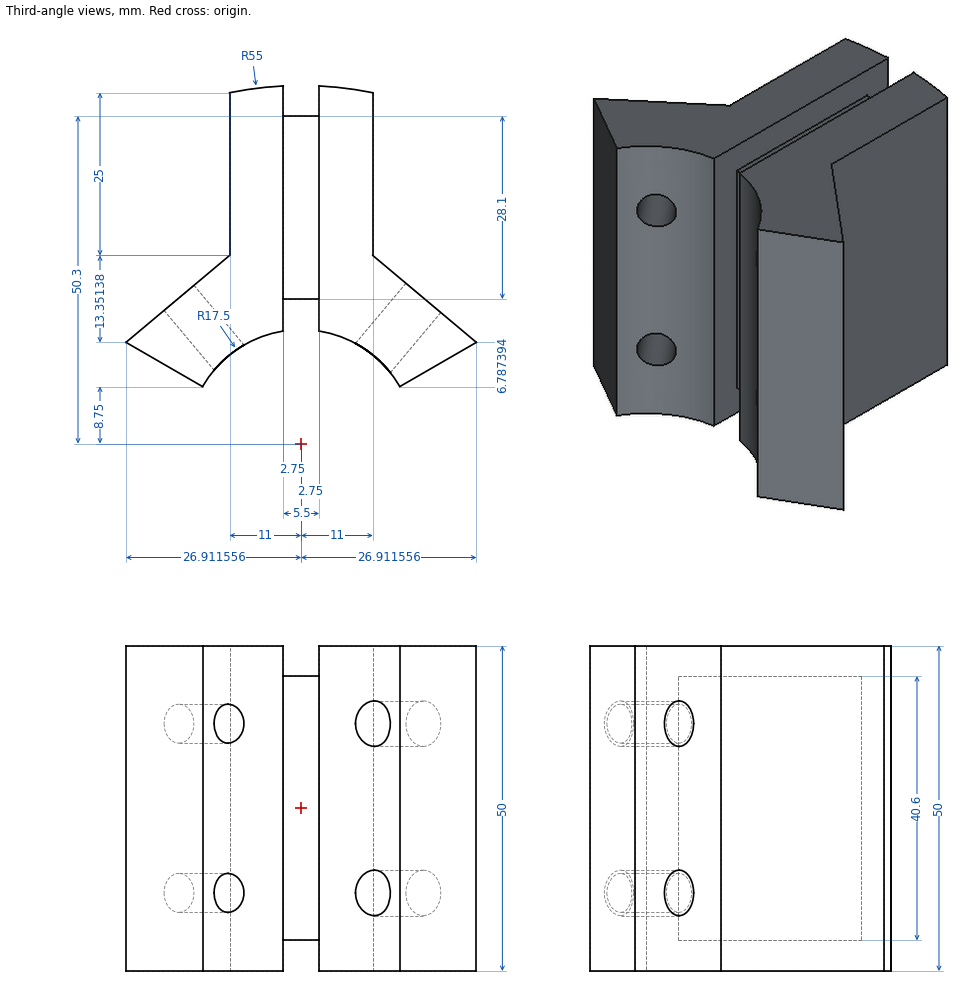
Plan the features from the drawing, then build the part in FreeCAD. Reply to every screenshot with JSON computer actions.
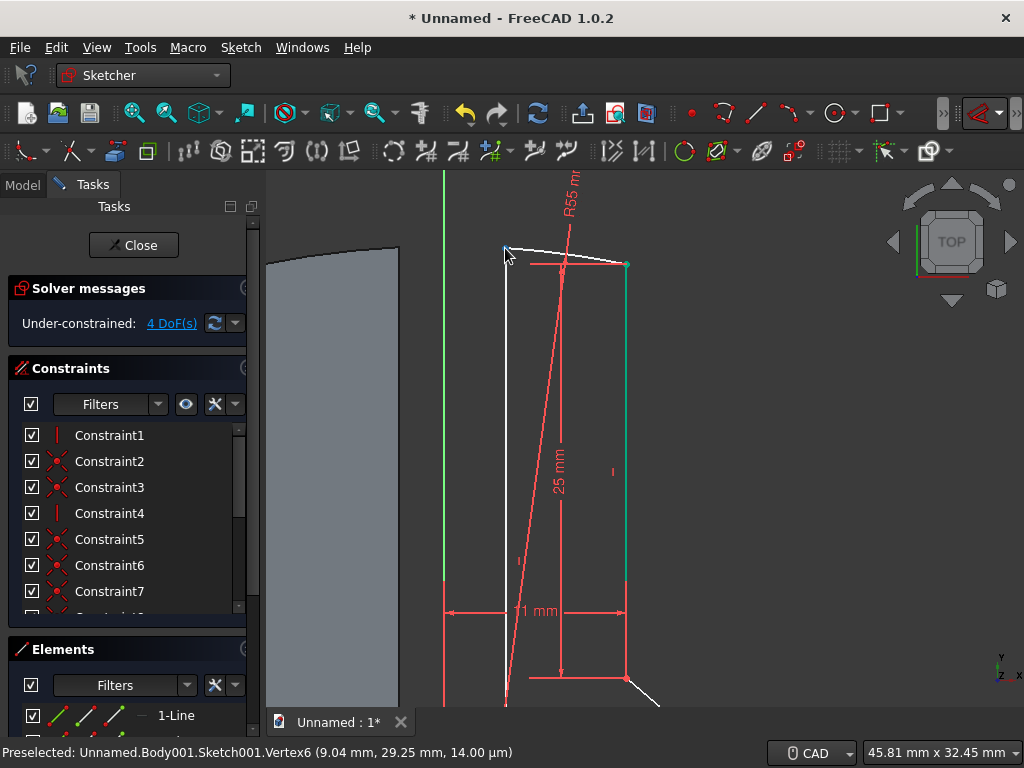
{"action": "left_click", "coordinate": [506, 248]}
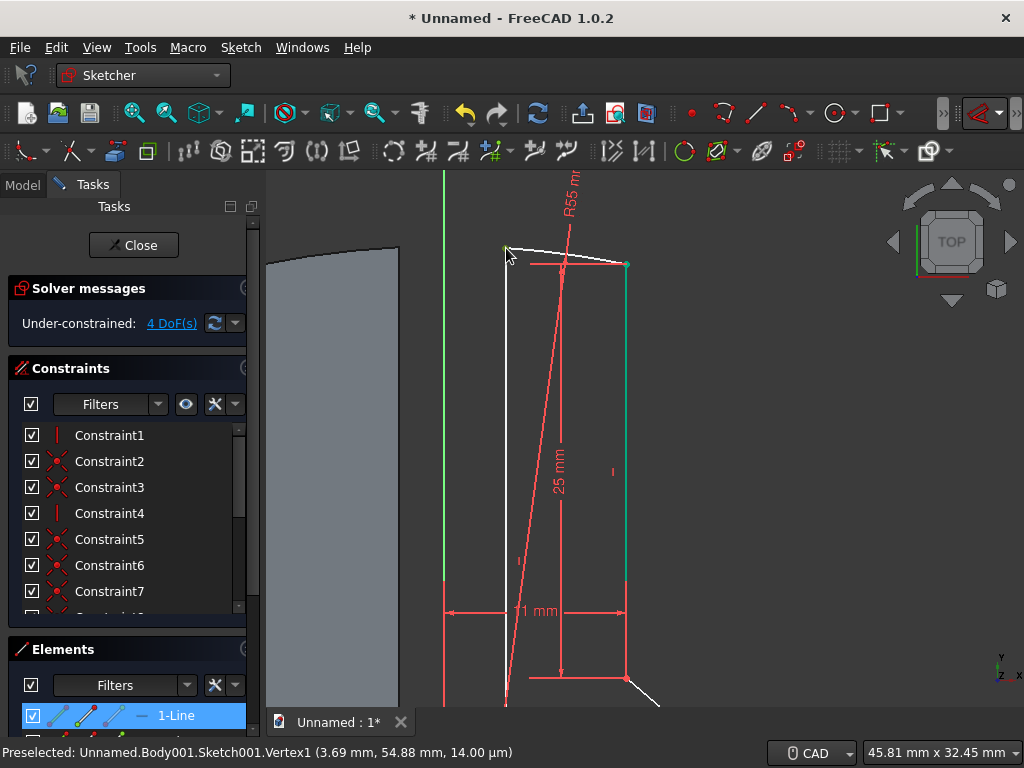
{"action": "key", "text": "l"}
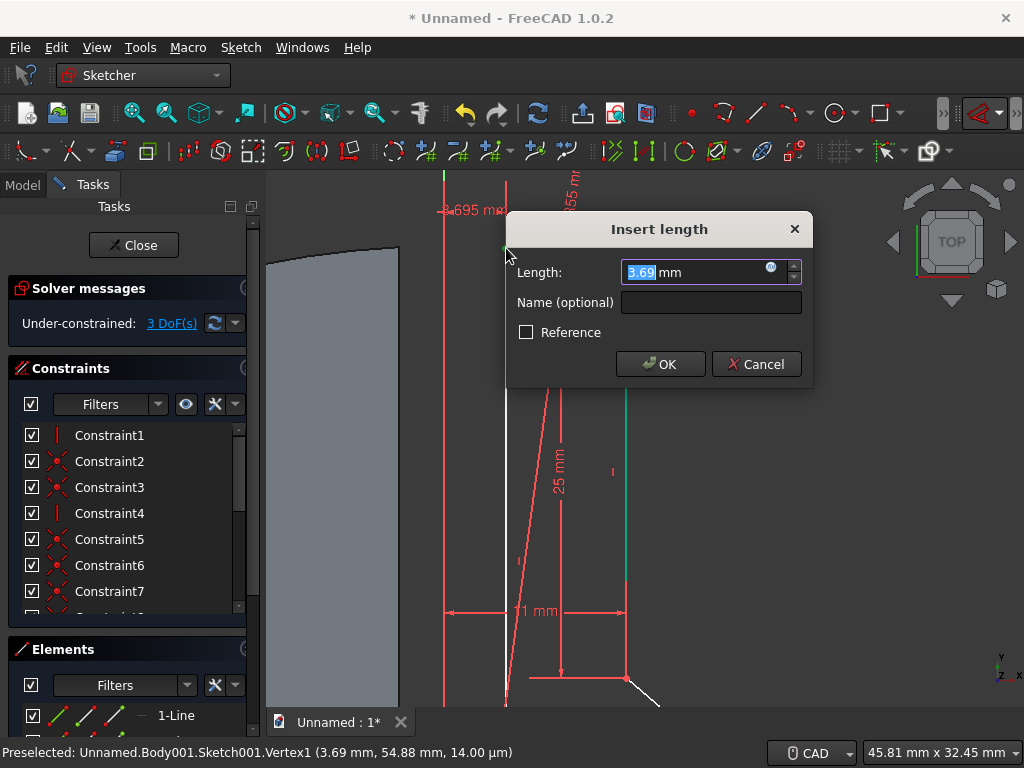
{"action": "type", "text": "2.75"}
{"action": "key", "text": "Return"}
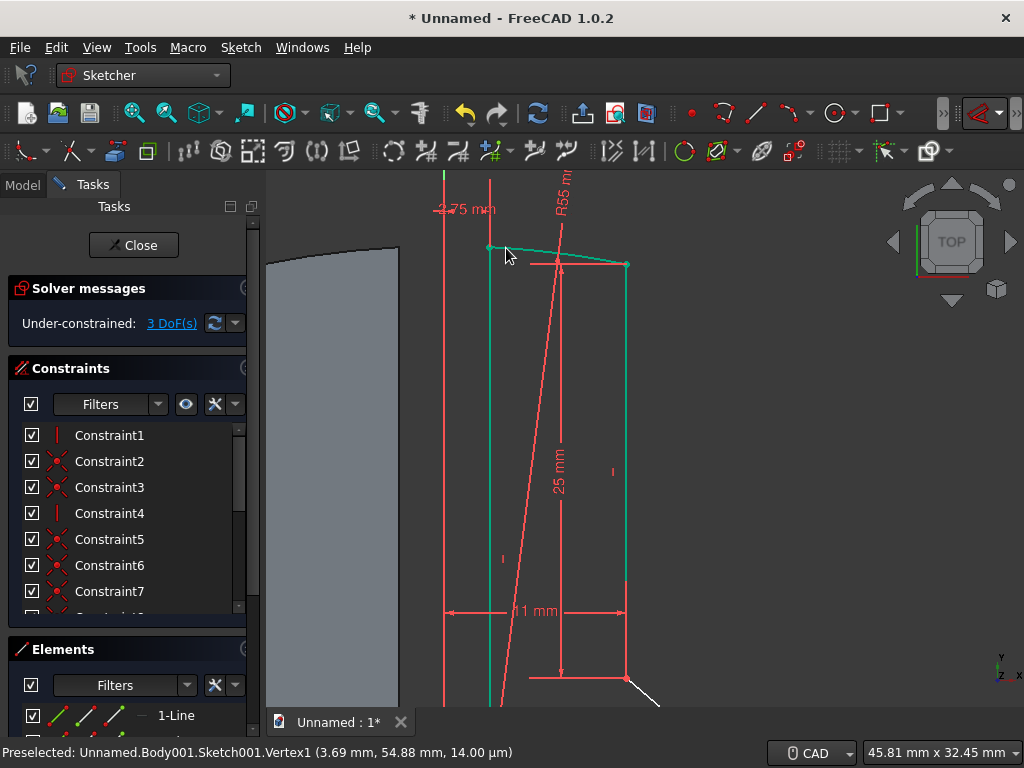
{"action": "scroll", "coordinate": [524, 285], "scroll_direction": "down", "scroll_amount": 5}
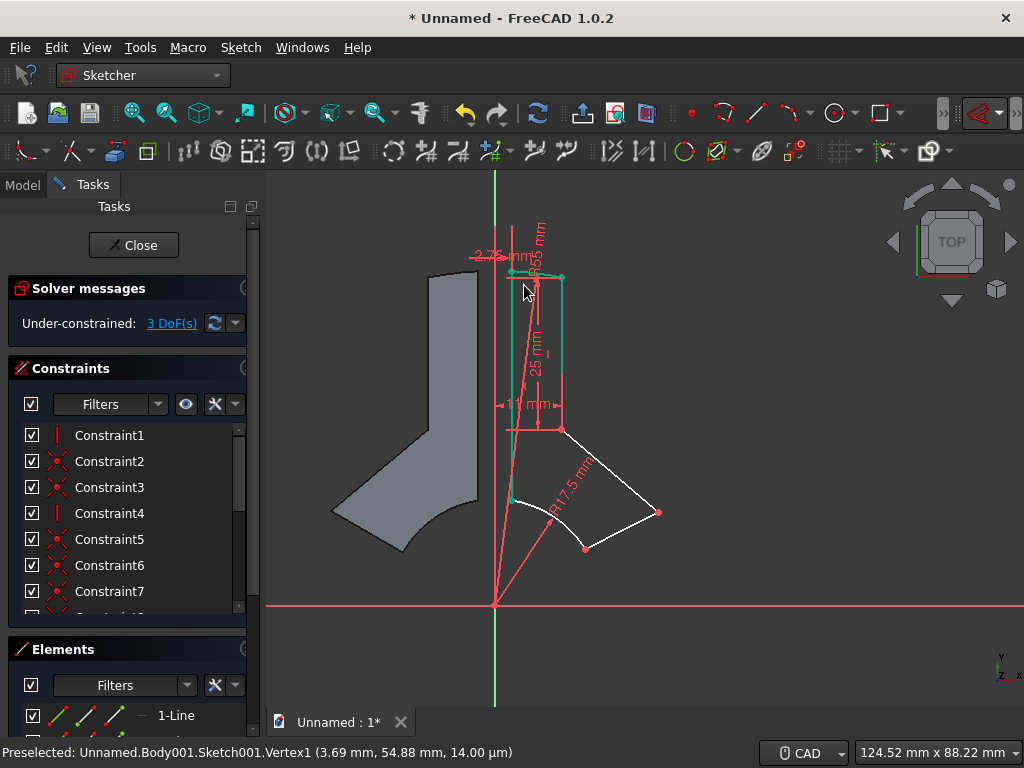
{"action": "left_click", "coordinate": [585, 549]}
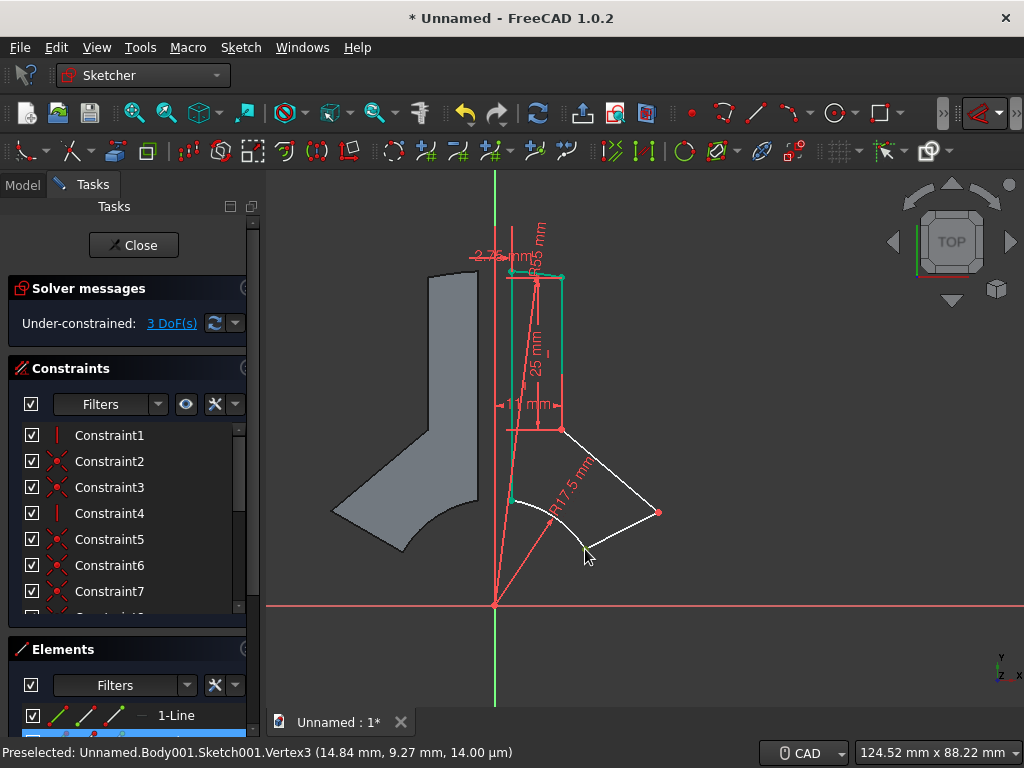
{"action": "left_click", "coordinate": [1002, 114]}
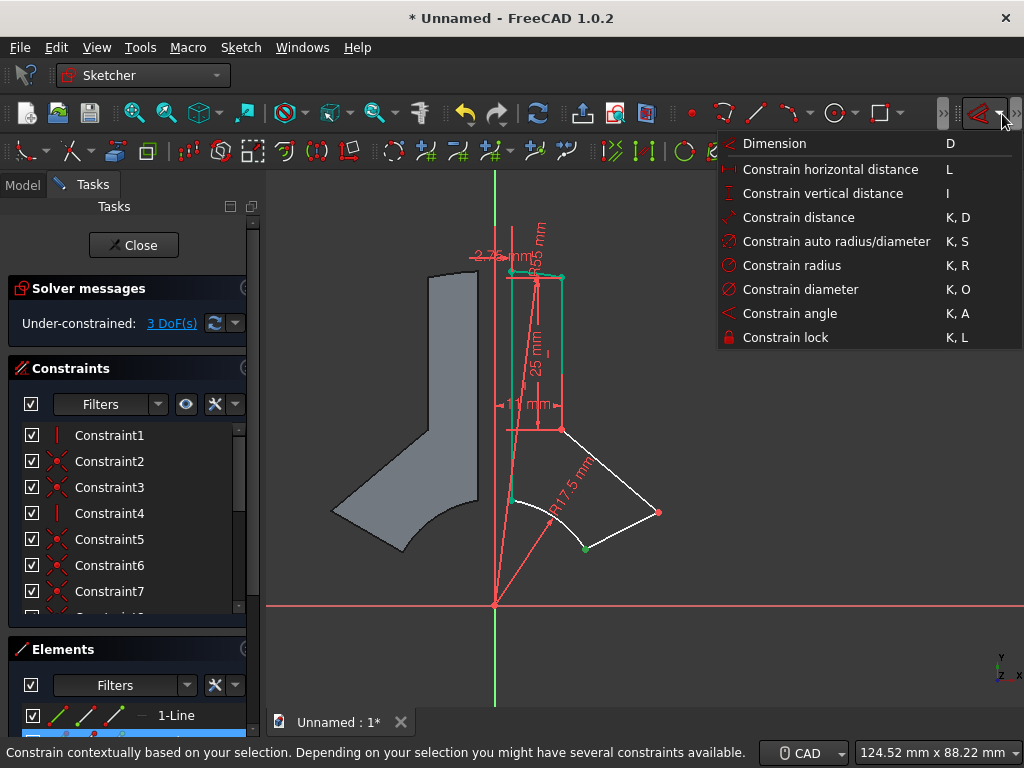
{"action": "left_click", "coordinate": [870, 193]}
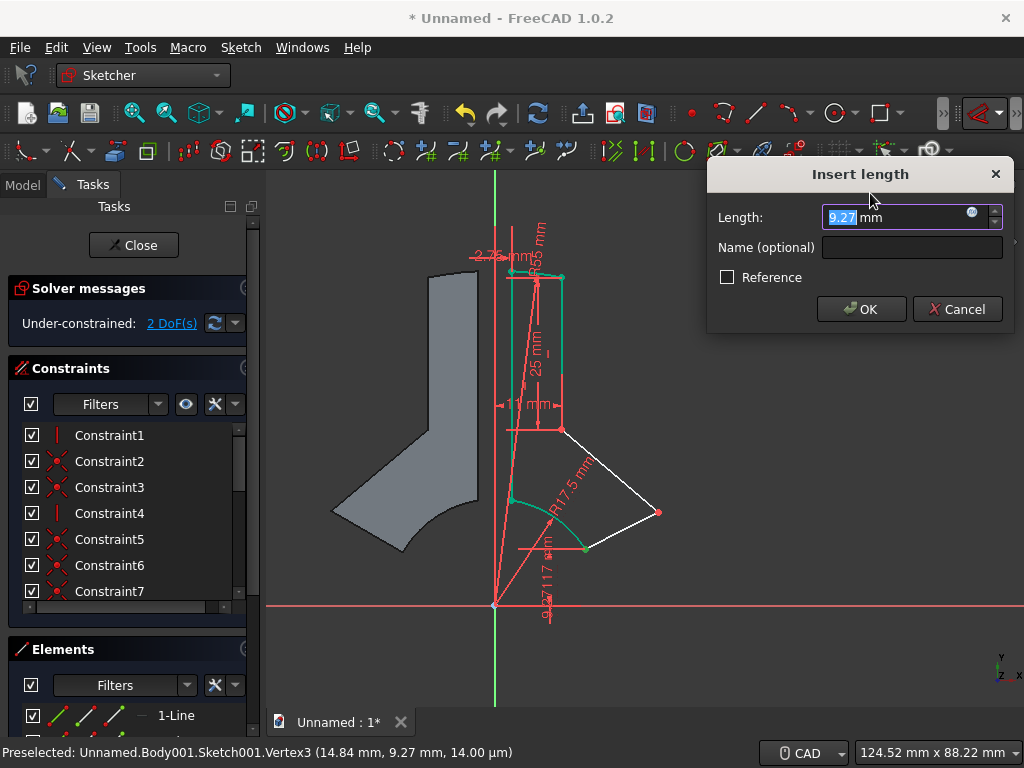
{"action": "type", "text": "8.75"}
{"action": "key", "text": "Return"}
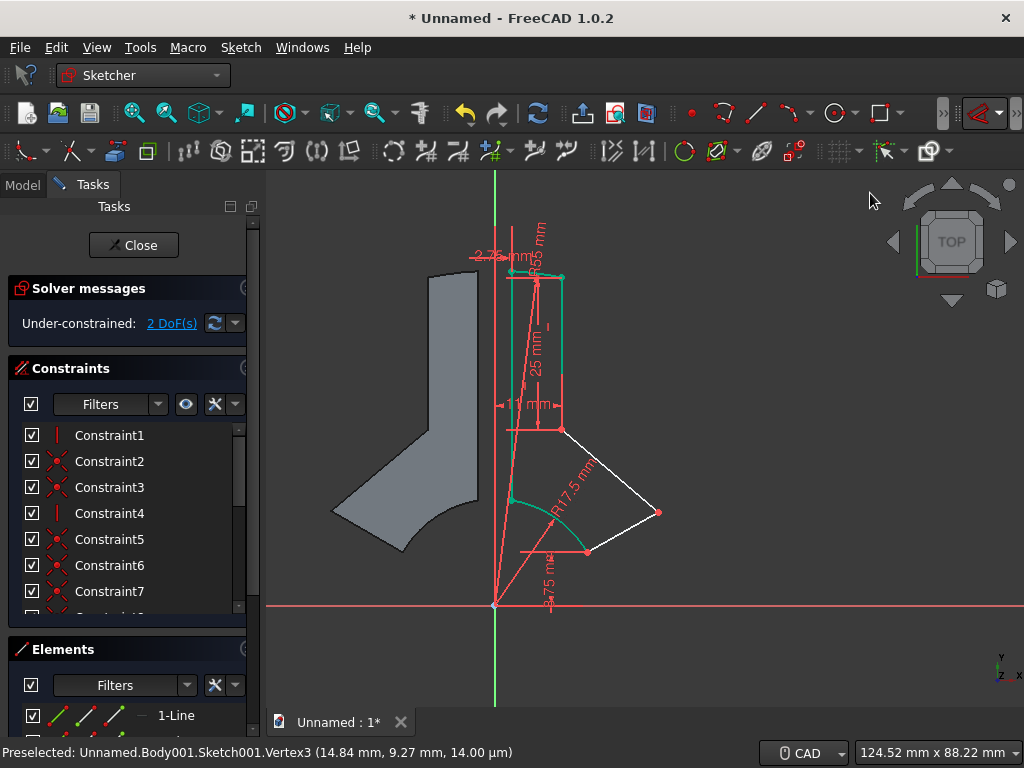
{"action": "left_click", "coordinate": [609, 540]}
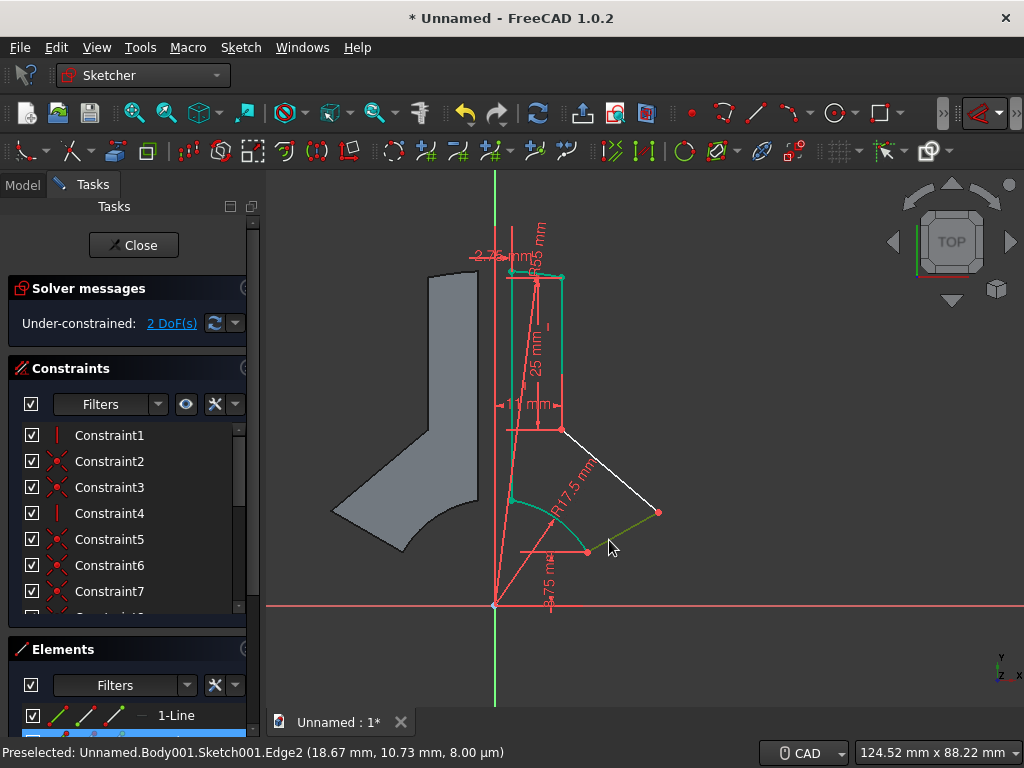
{"action": "left_click", "coordinate": [1002, 114]}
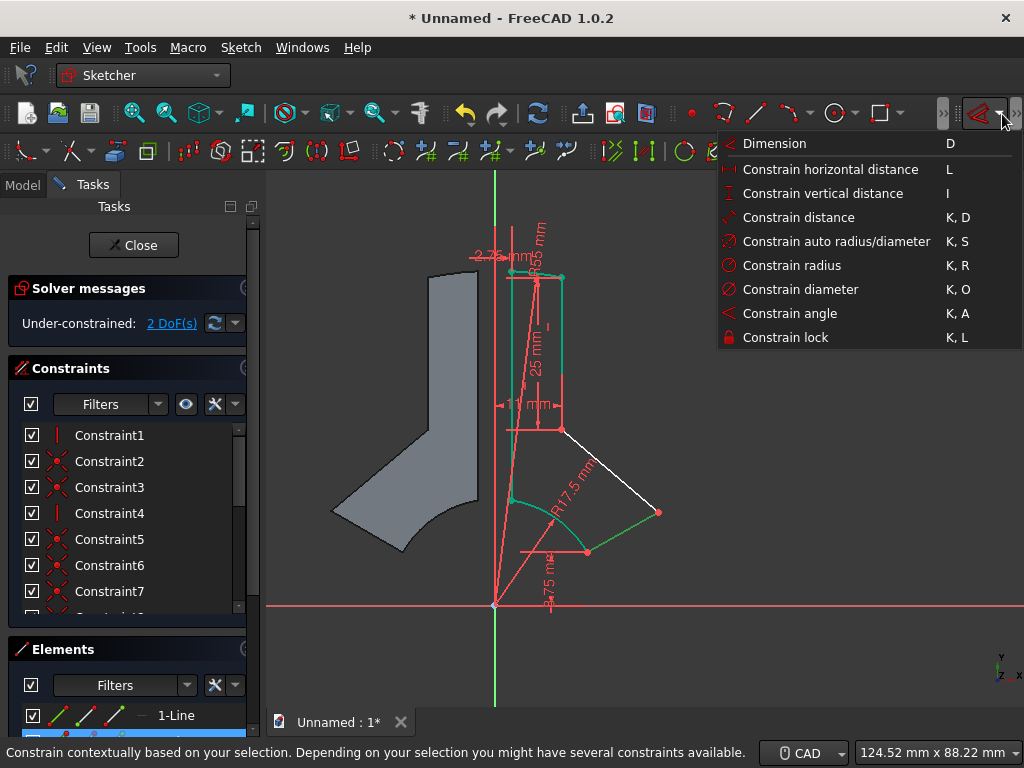
{"action": "left_click", "coordinate": [870, 193]}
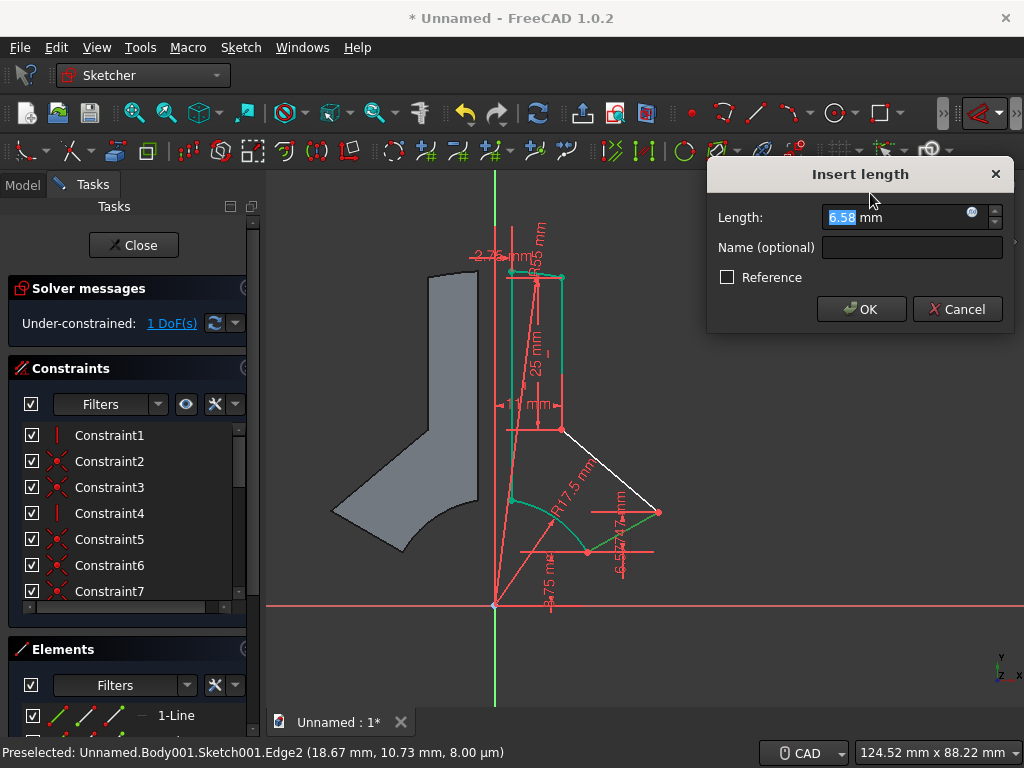
{"action": "type", "text": "6.787394"}
{"action": "key", "text": "Return"}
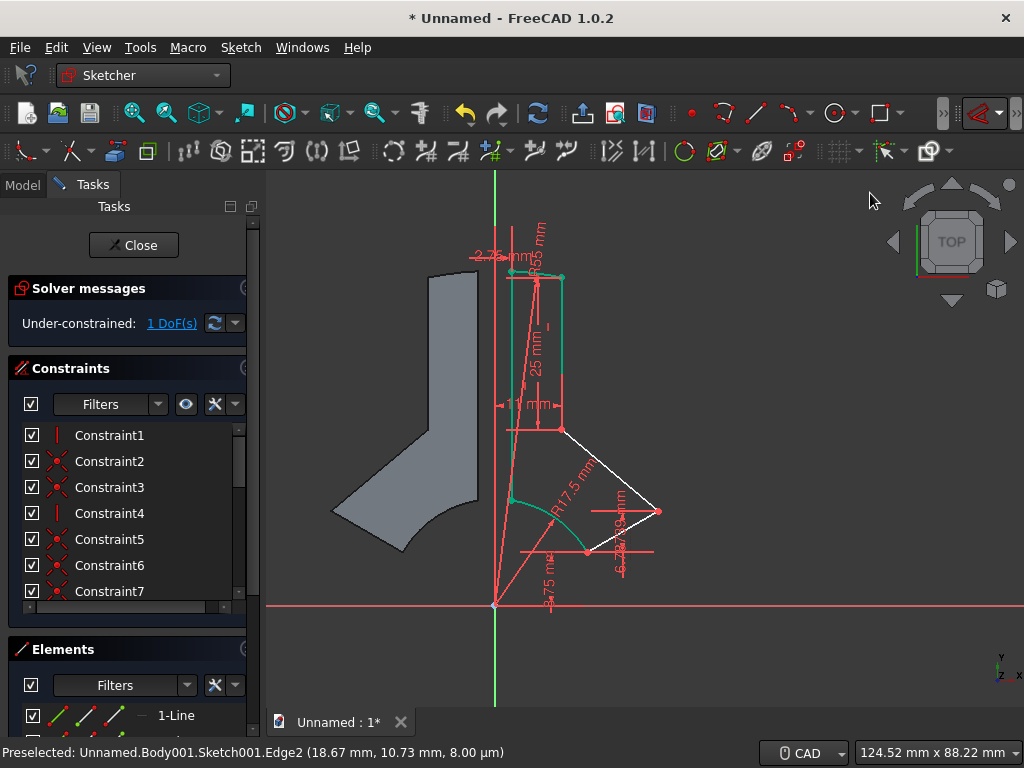
{"action": "left_click", "coordinate": [658, 511]}